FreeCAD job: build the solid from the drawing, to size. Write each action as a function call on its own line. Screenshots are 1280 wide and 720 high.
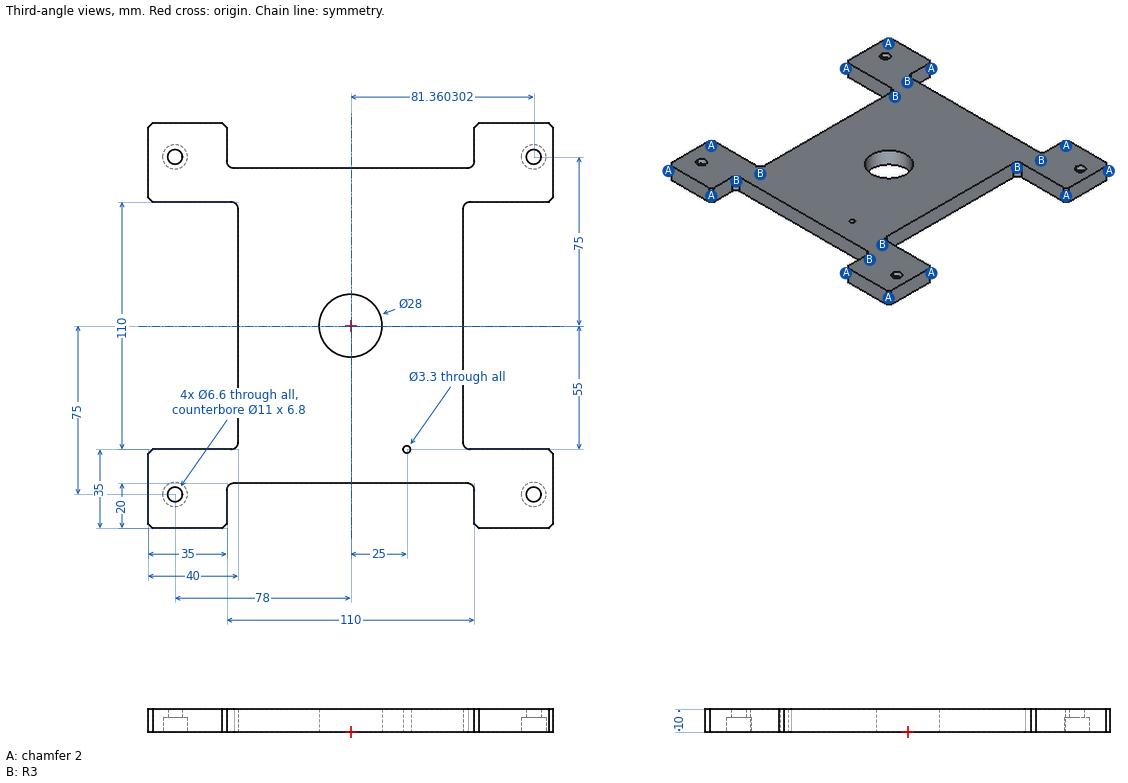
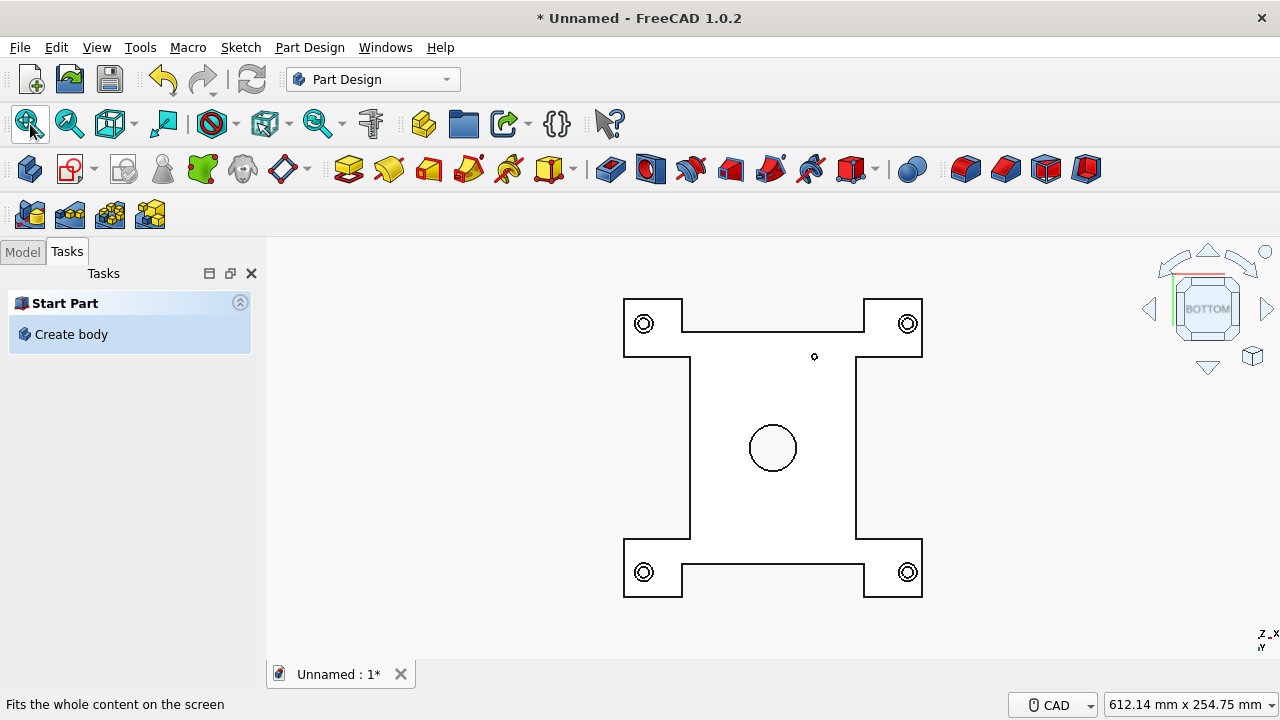
key(0)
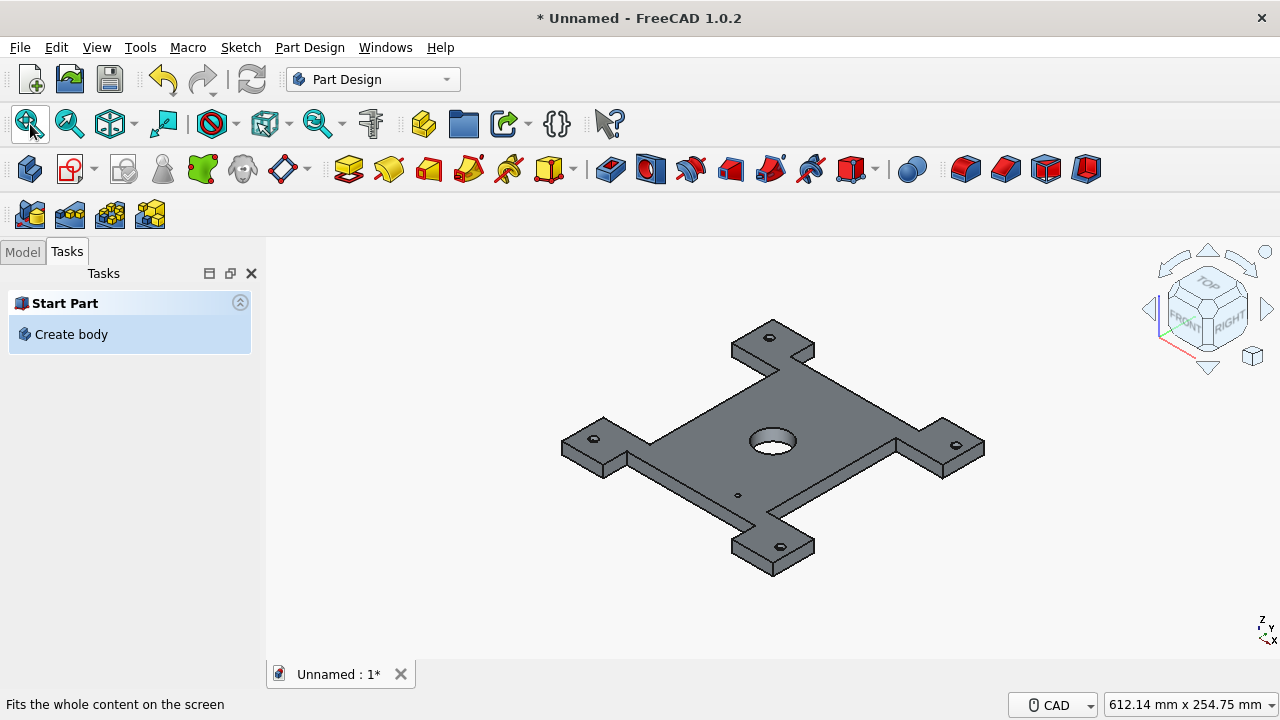
click(943, 471)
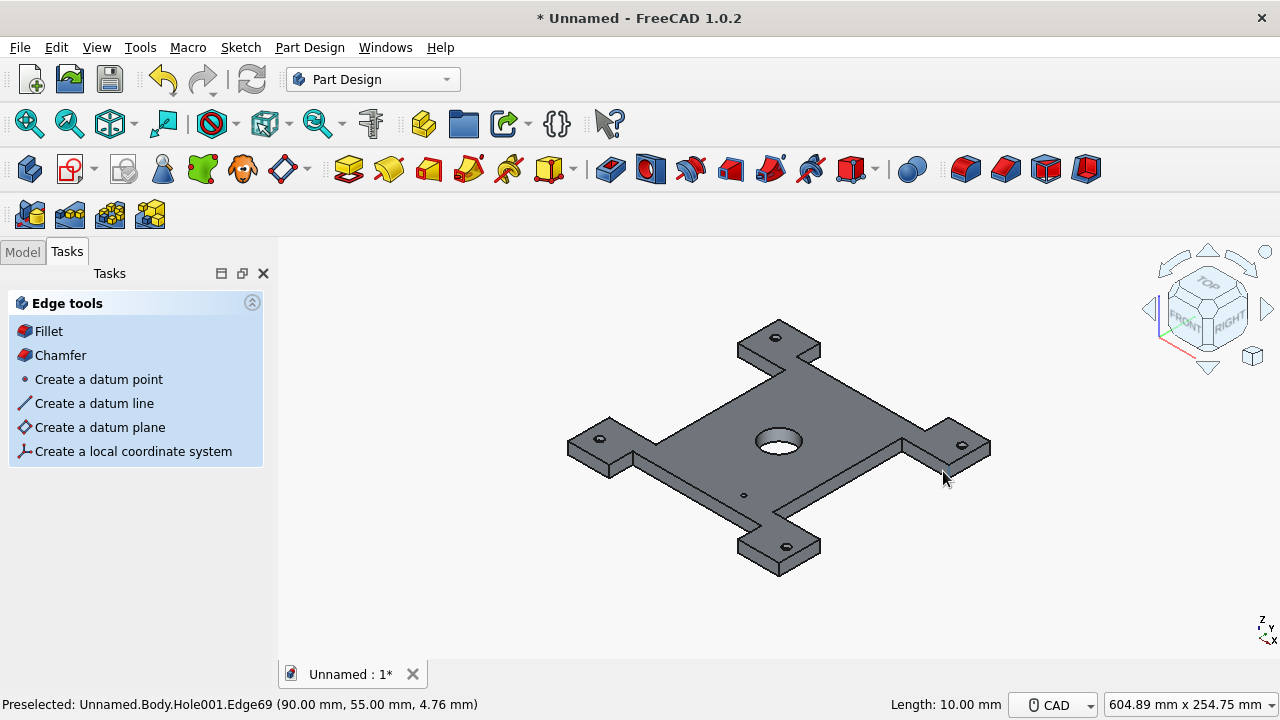
click(779, 569, ctrl)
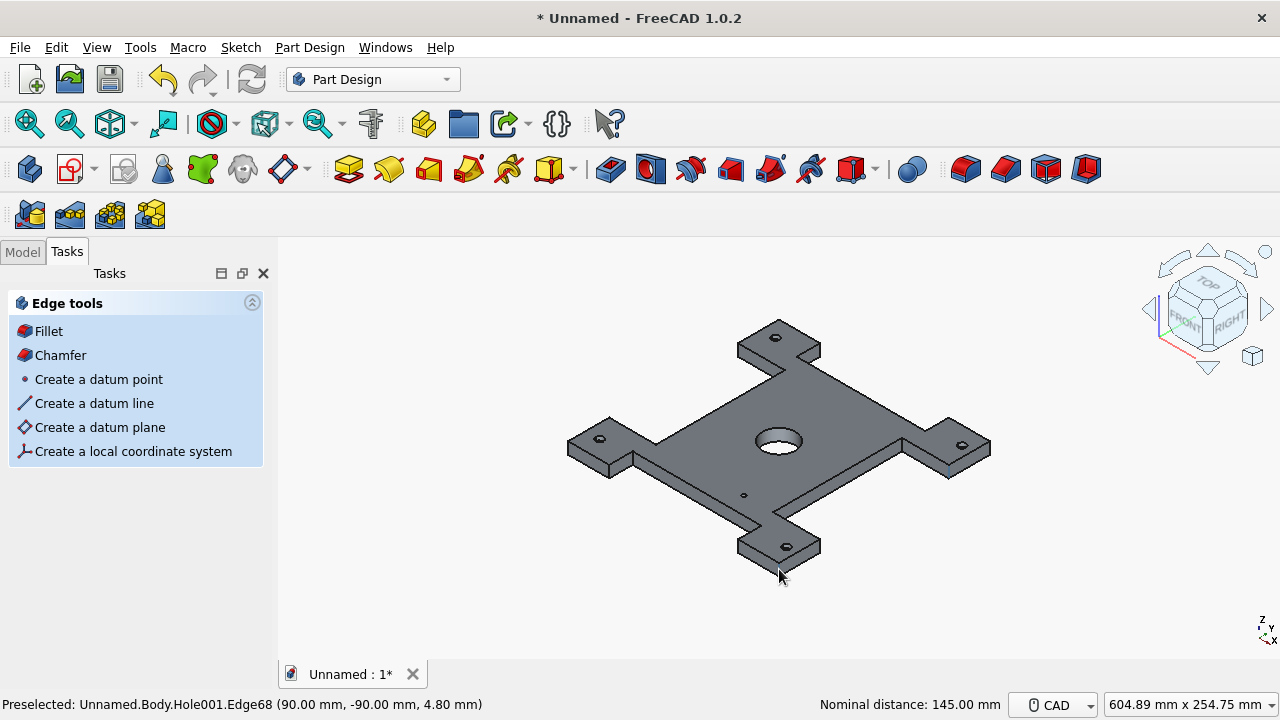
click(609, 471, ctrl)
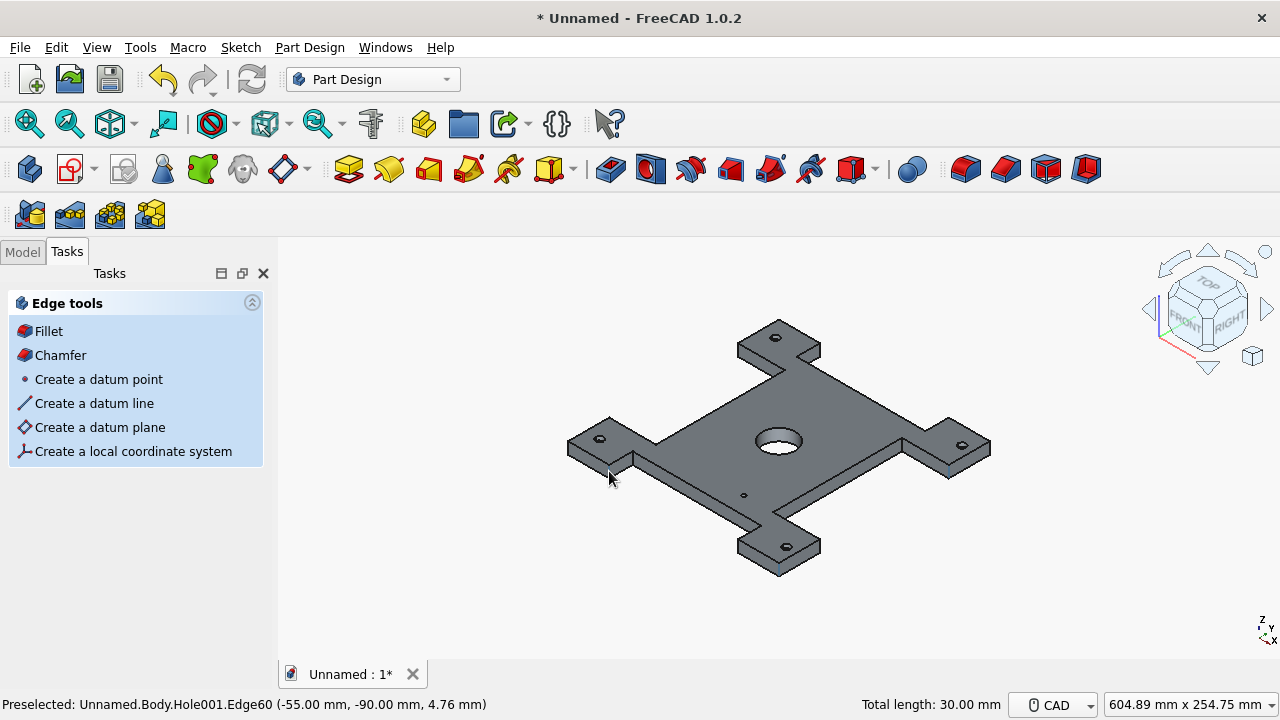
scroll(738, 349, up, 5)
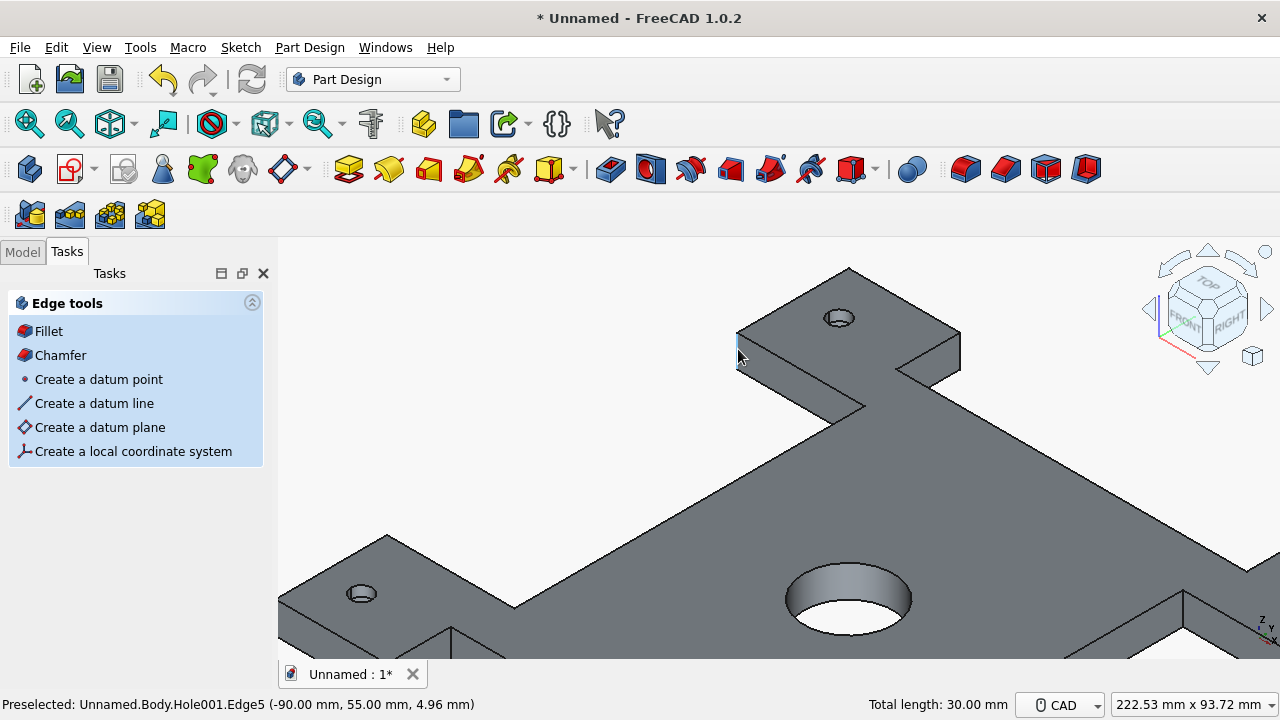
click(30, 124)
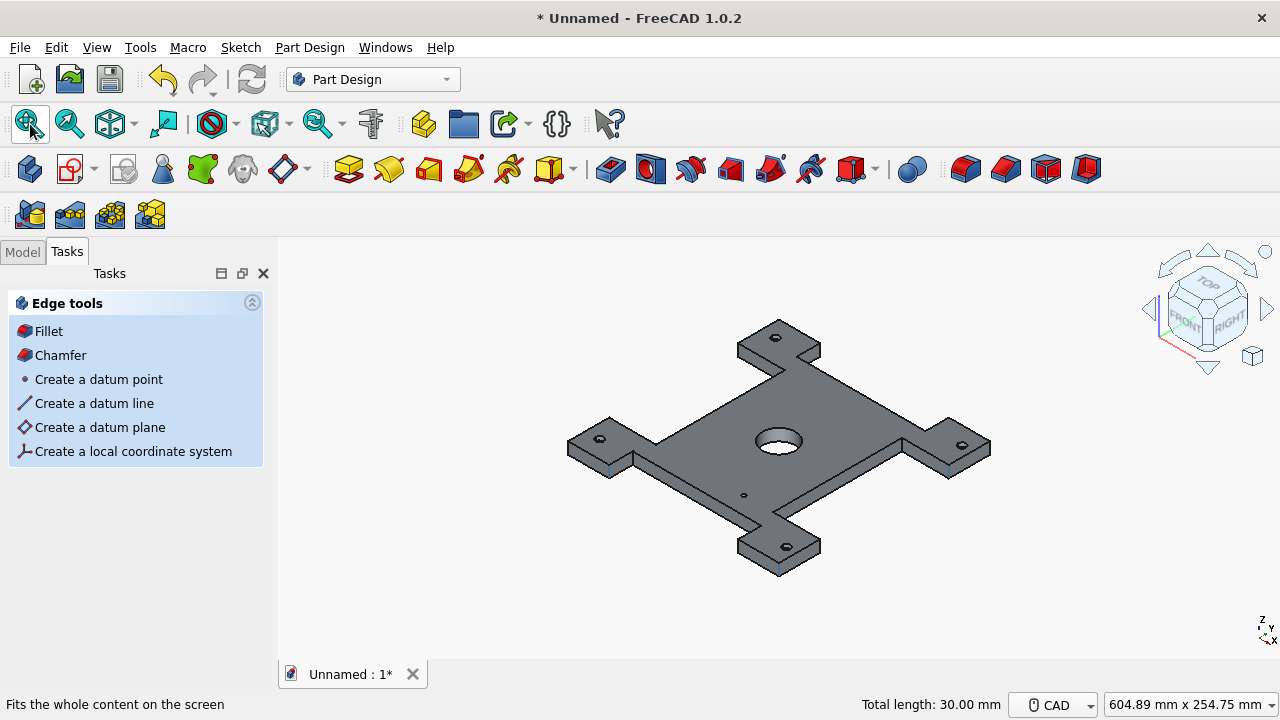
key(2)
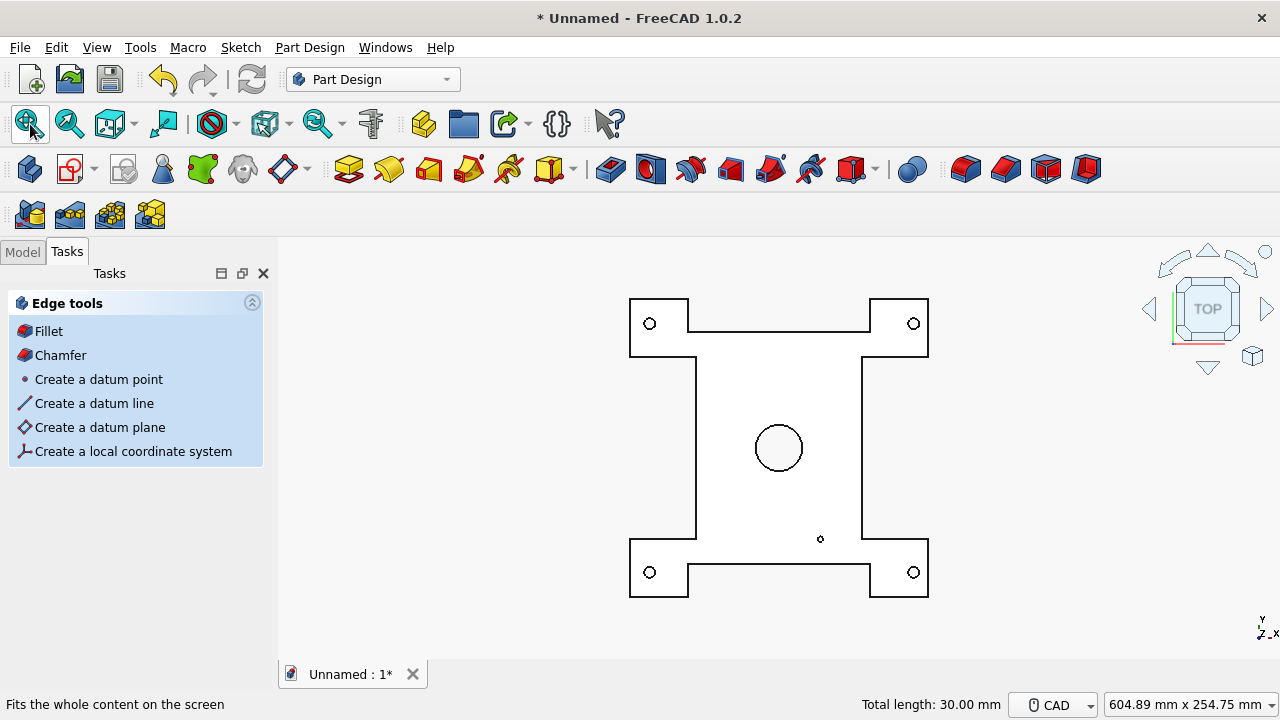
scroll(630, 356, up, 5)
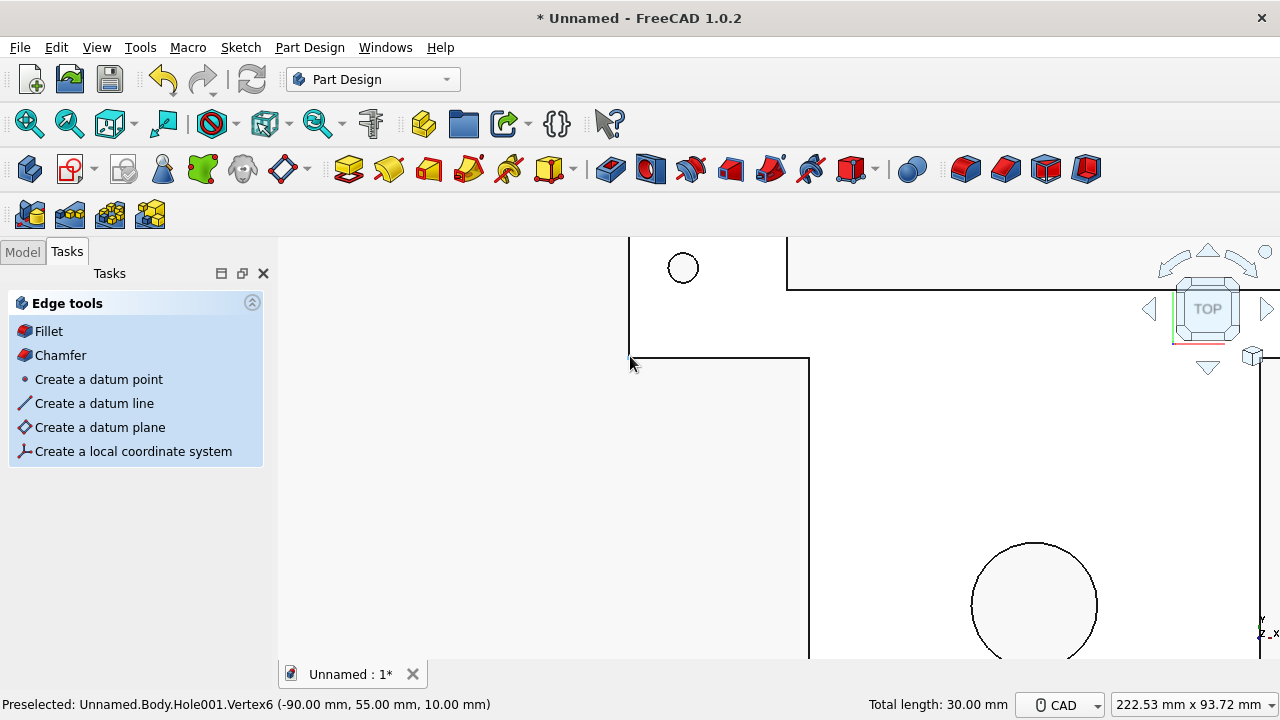
click(30, 124)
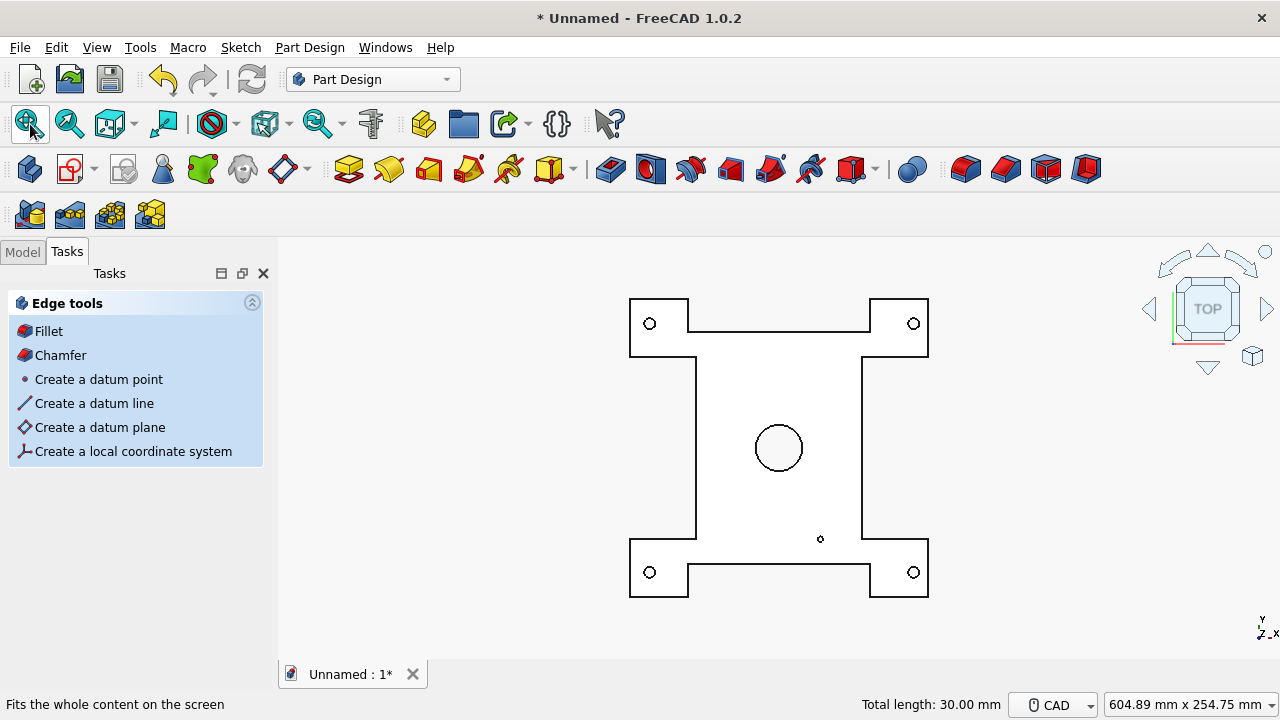
key(1)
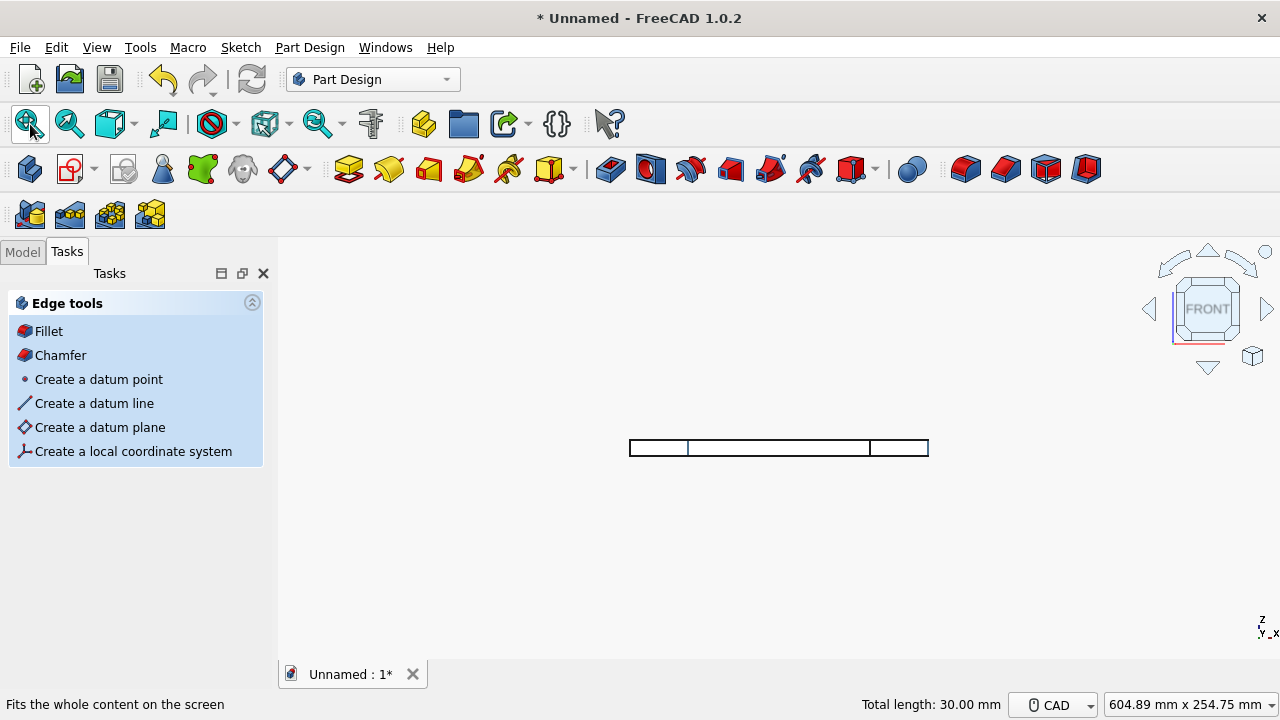
click(30, 124)